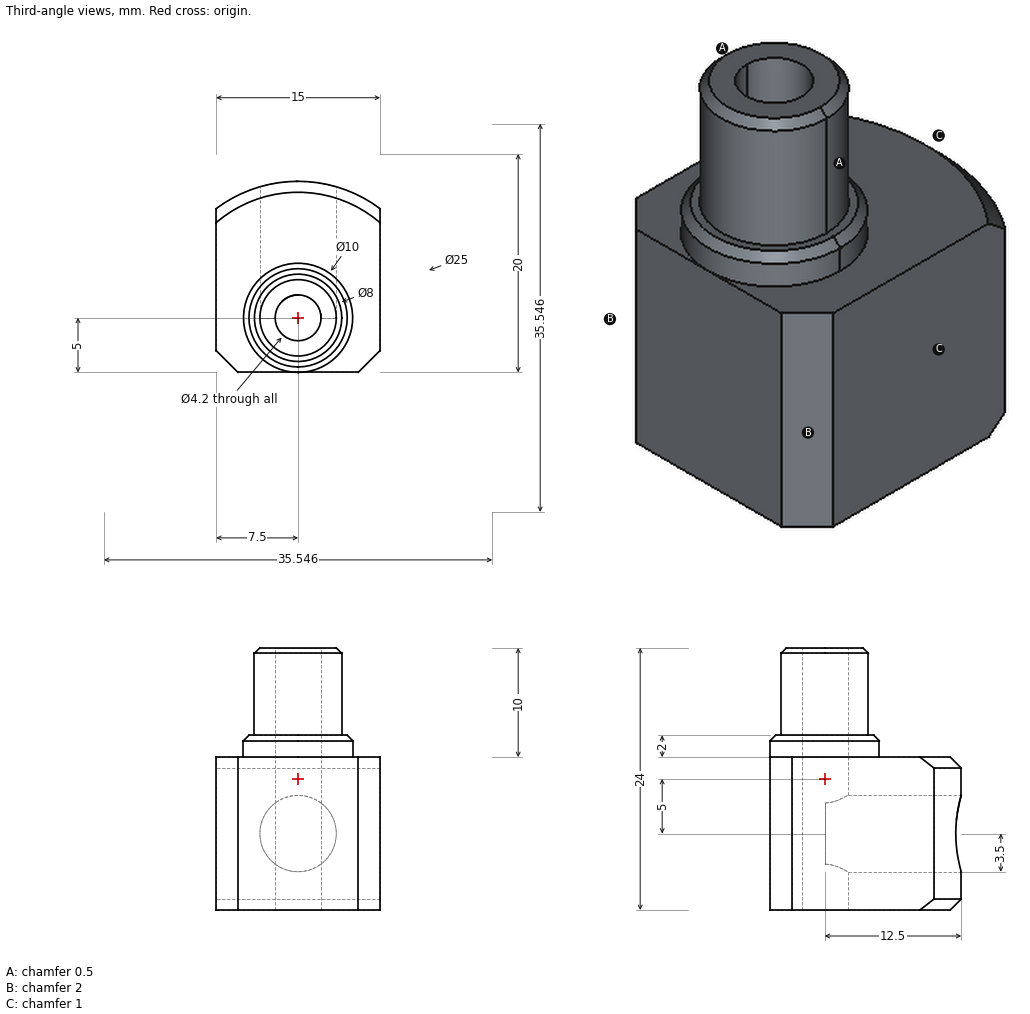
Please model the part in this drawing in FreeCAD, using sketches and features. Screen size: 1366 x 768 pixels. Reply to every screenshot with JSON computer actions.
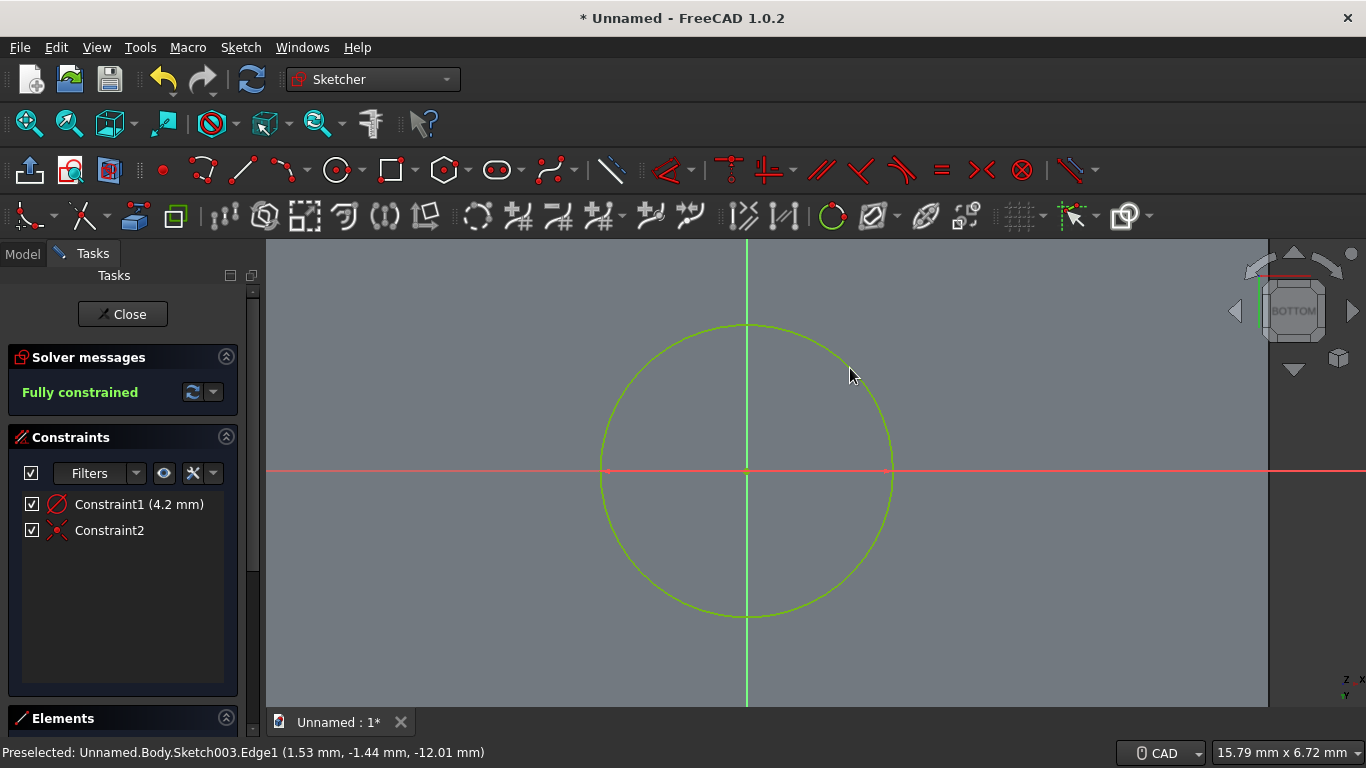
{"action": "left_click", "coordinate": [123, 314]}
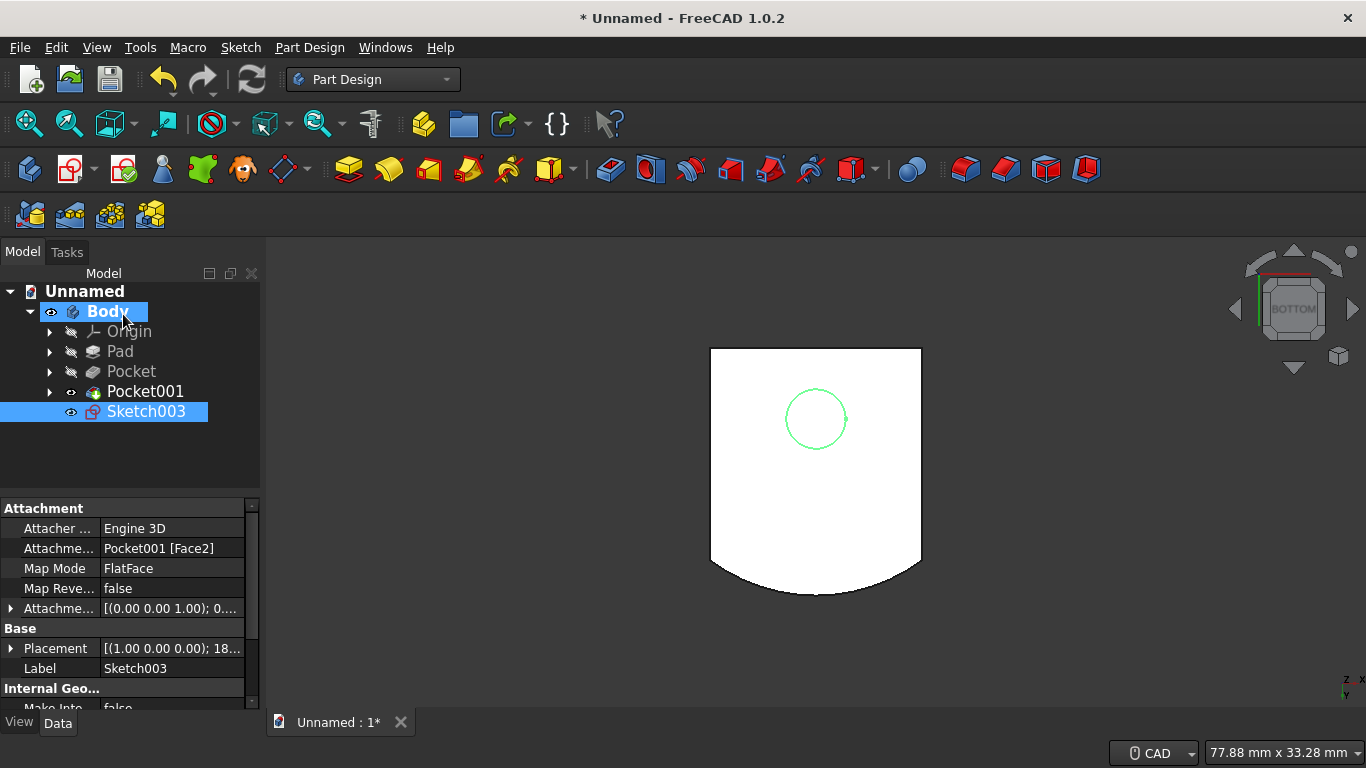
{"action": "left_click", "coordinate": [652, 170]}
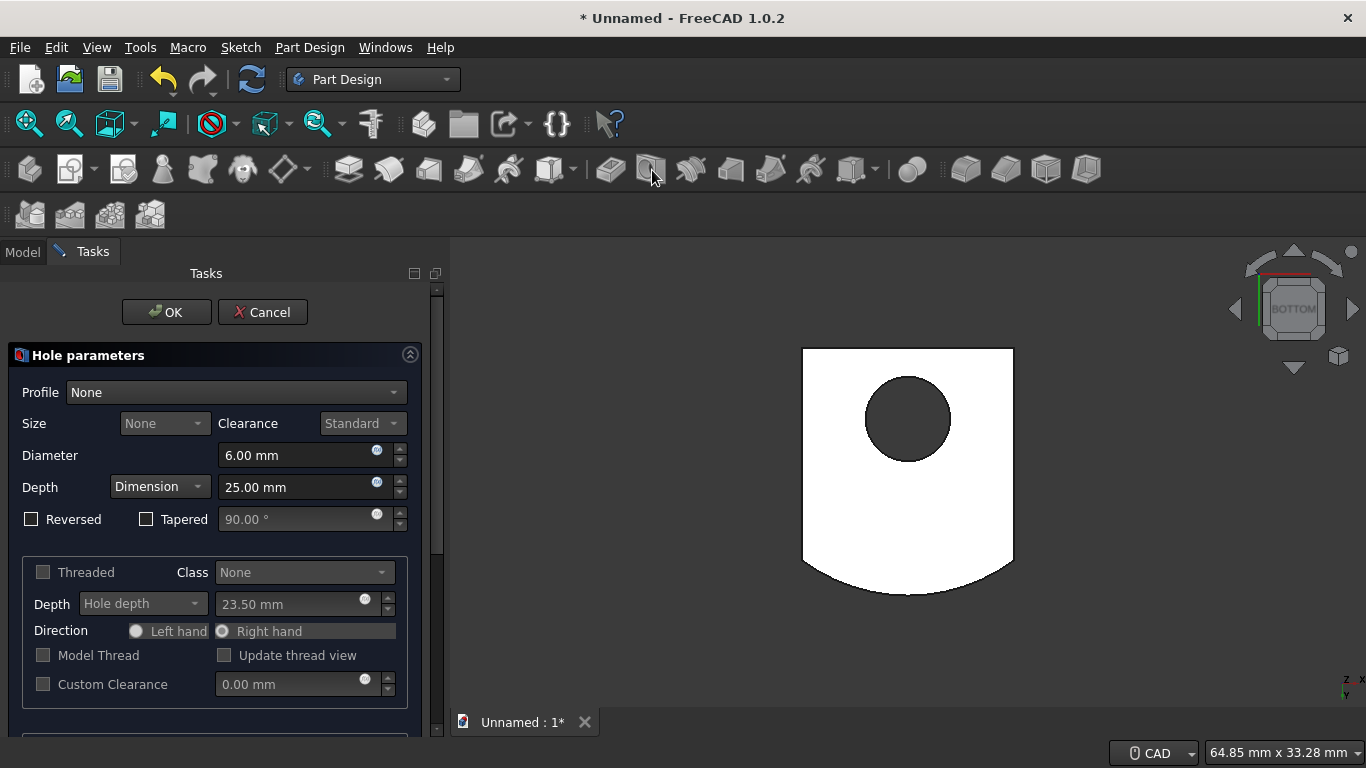
{"action": "triple_click", "coordinate": [305, 455]}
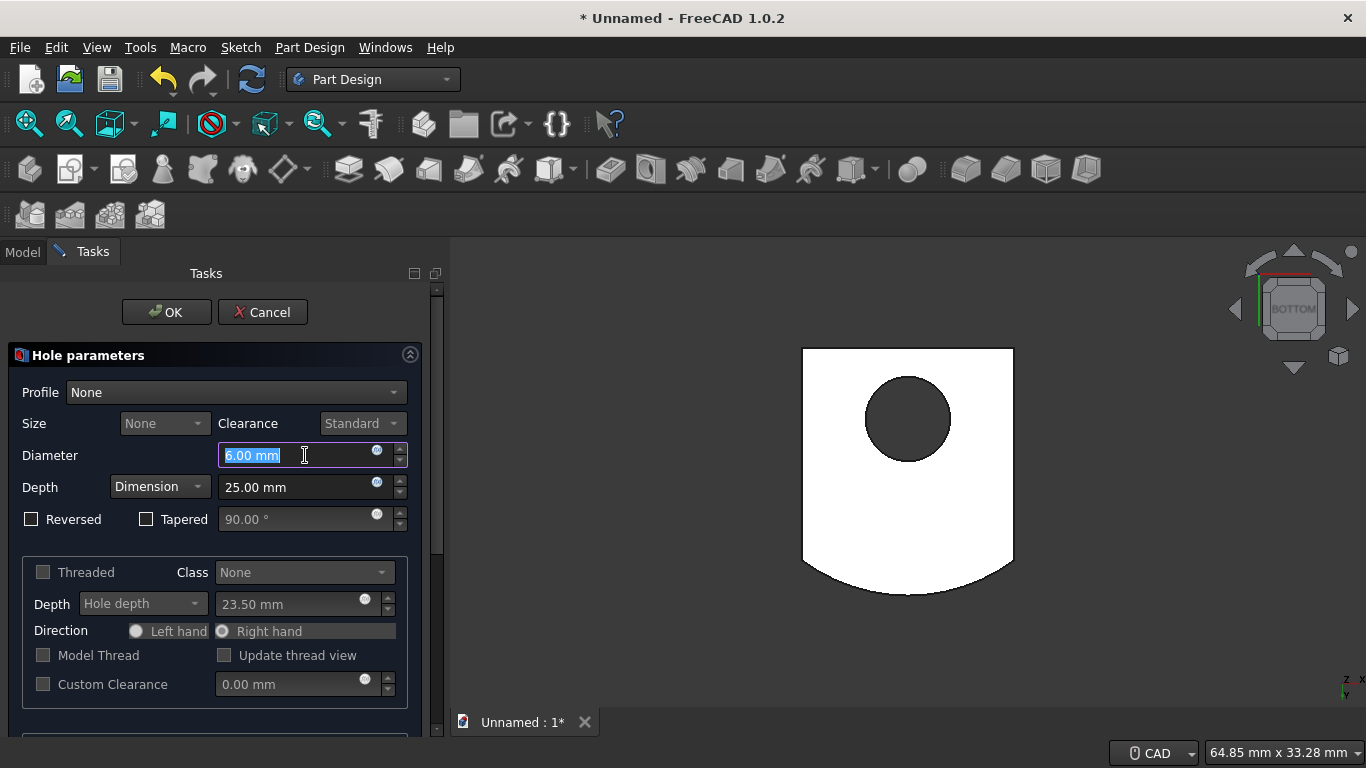
{"action": "type", "text": "4.2"}
{"action": "key", "text": "Tab"}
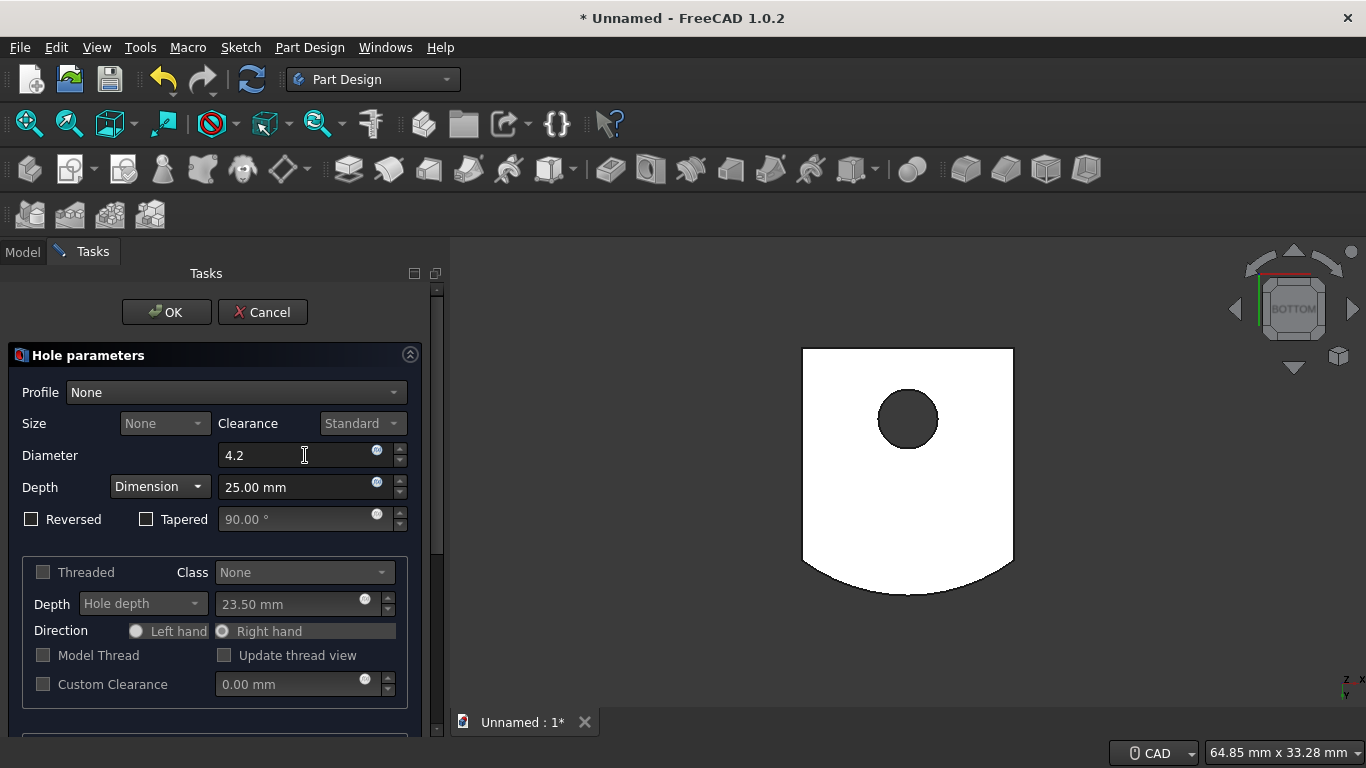
{"action": "left_click", "coordinate": [161, 486]}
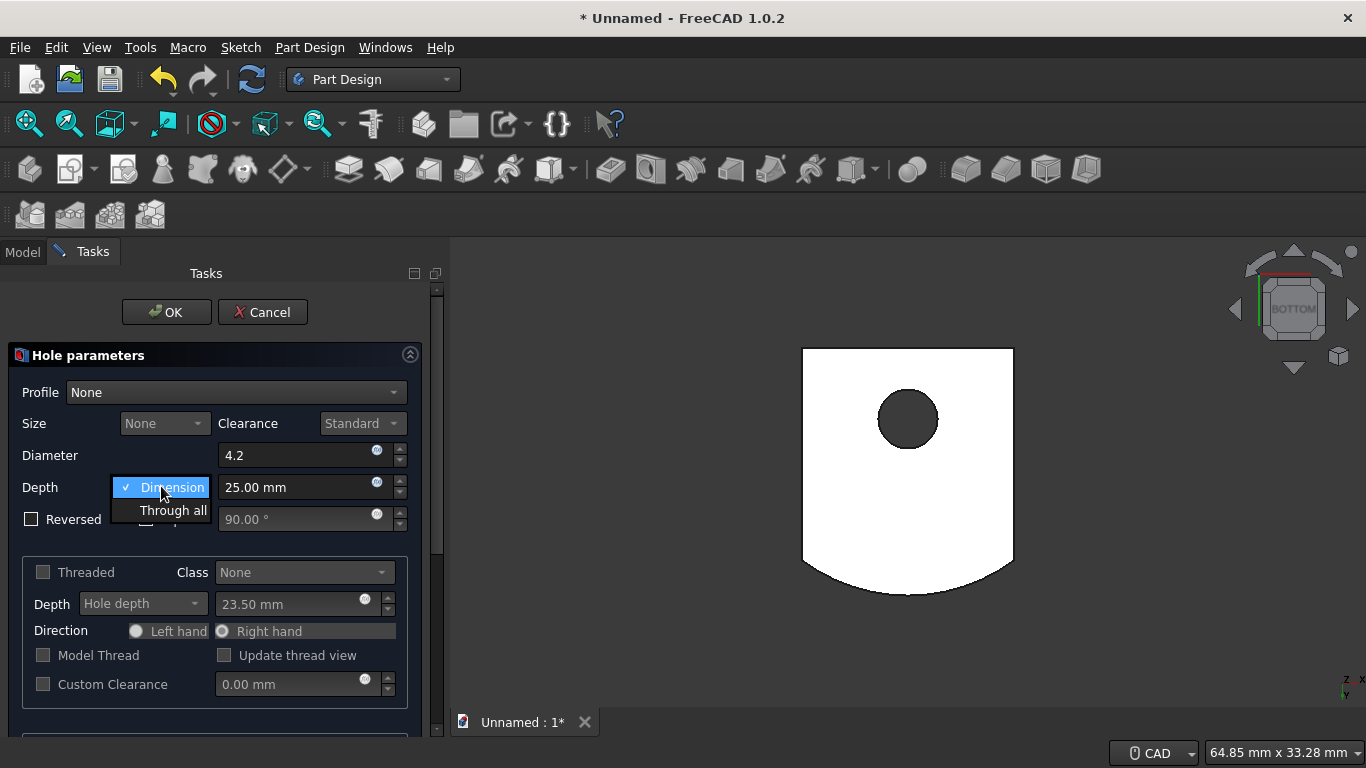
{"action": "left_click", "coordinate": [160, 510]}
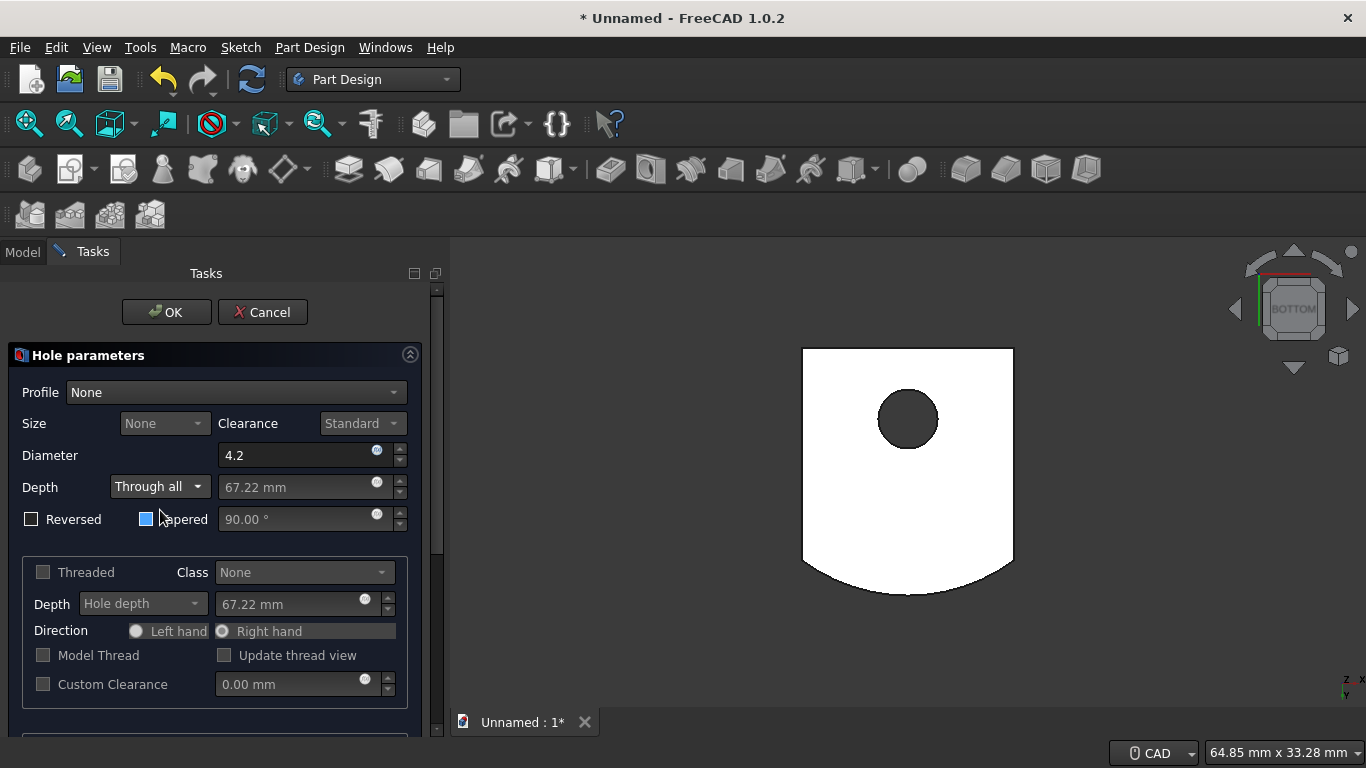
{"action": "left_click", "coordinate": [167, 312]}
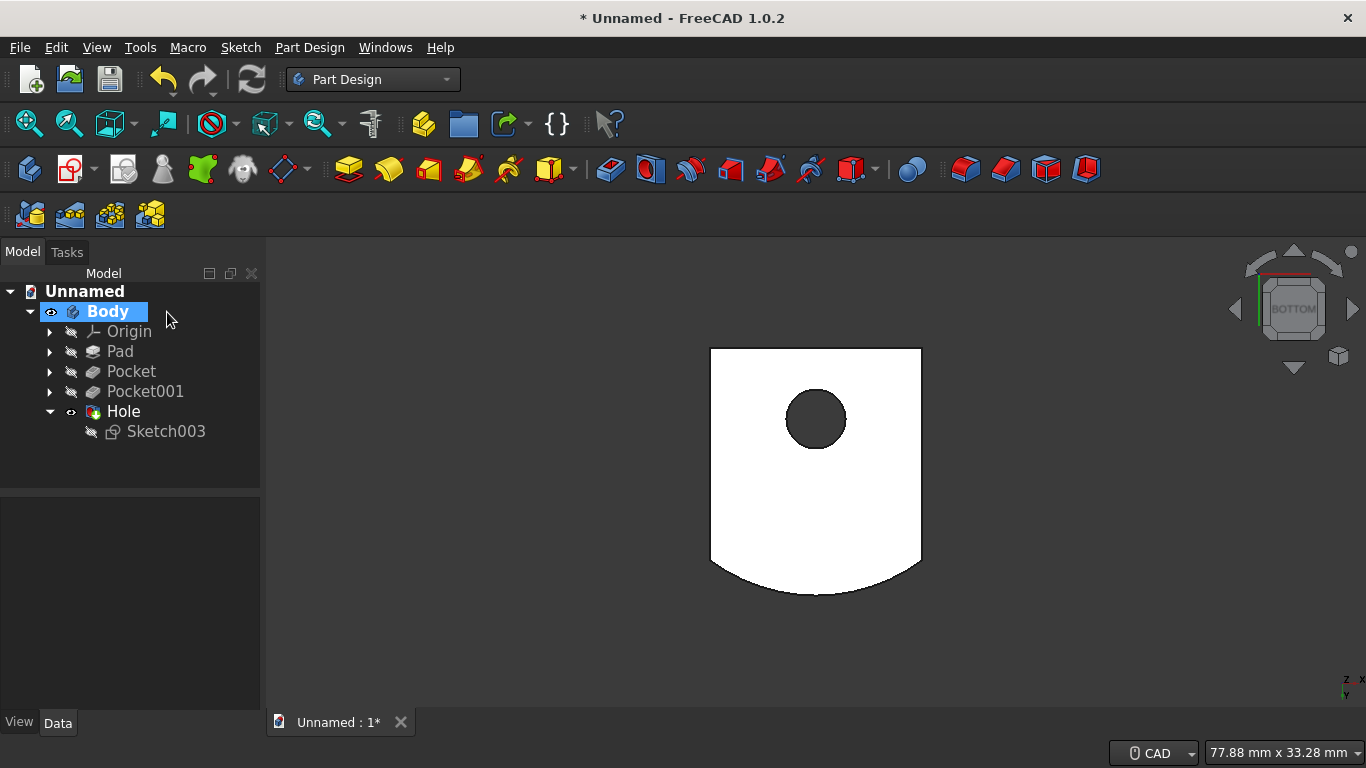
{"action": "left_click", "coordinate": [50, 332]}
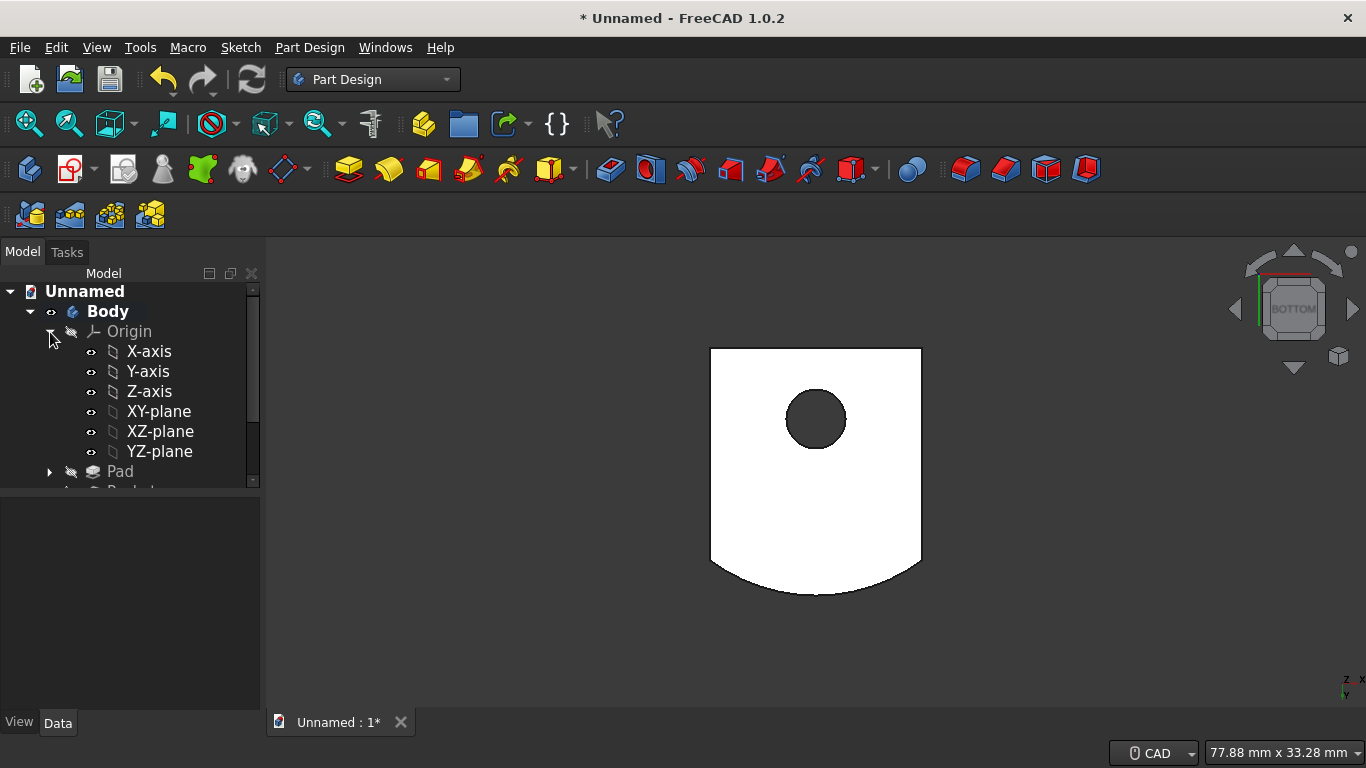
{"action": "left_click", "coordinate": [136, 412]}